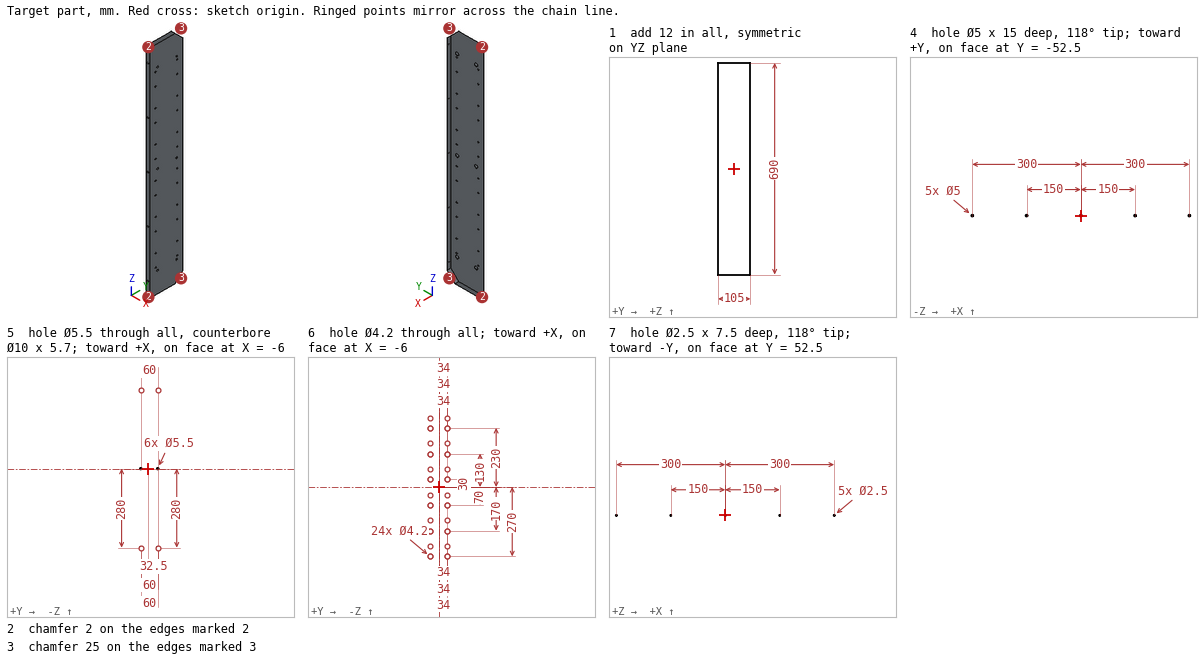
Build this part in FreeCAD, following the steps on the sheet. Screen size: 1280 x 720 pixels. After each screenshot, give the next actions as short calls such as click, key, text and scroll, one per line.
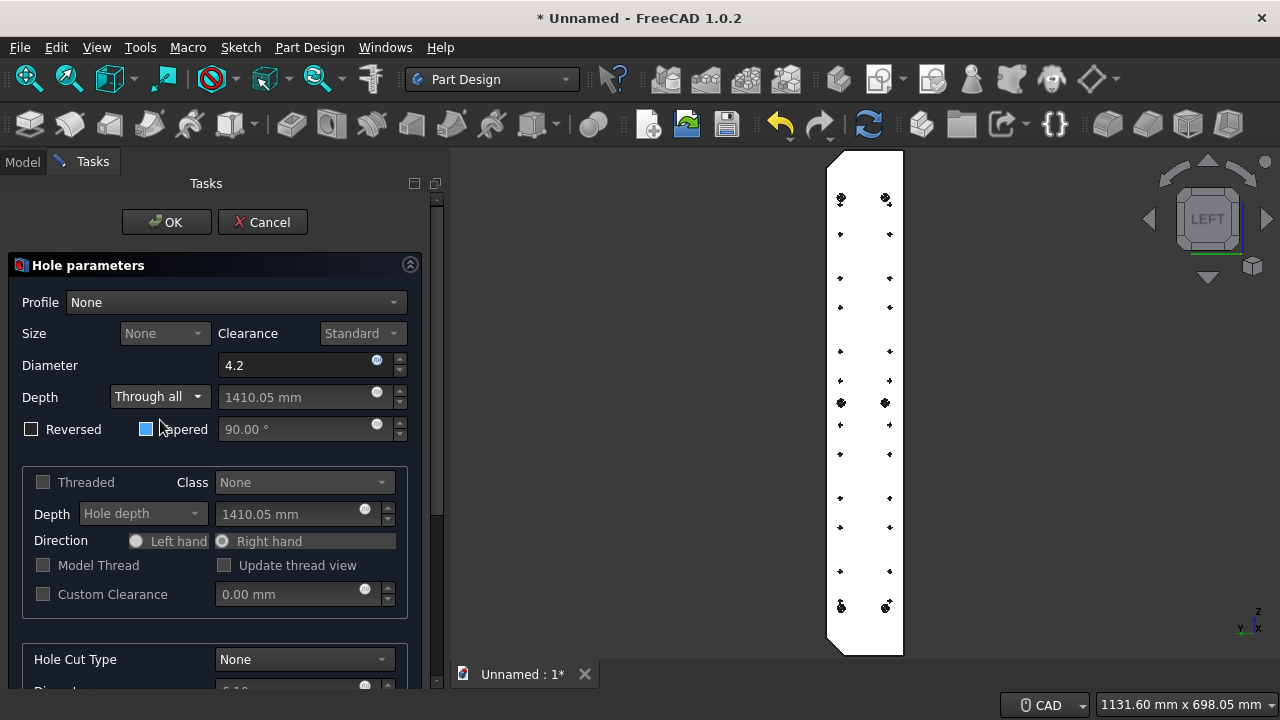
click(167, 222)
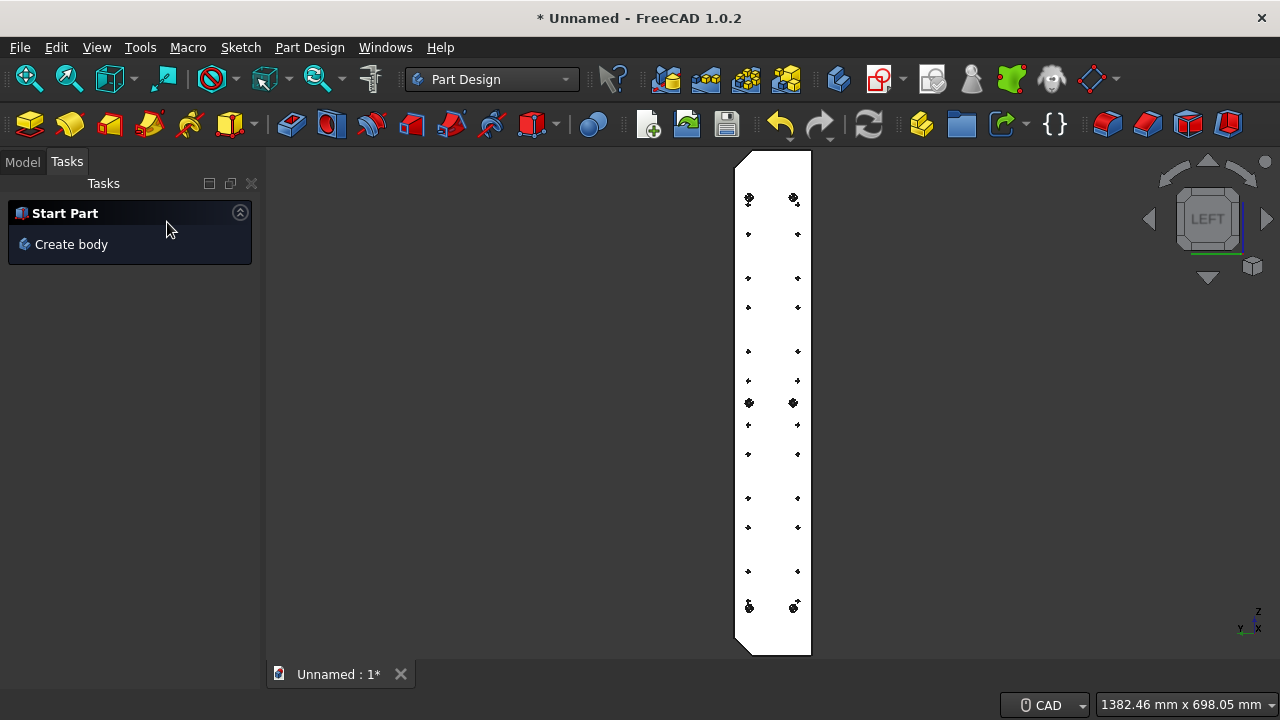
key(4)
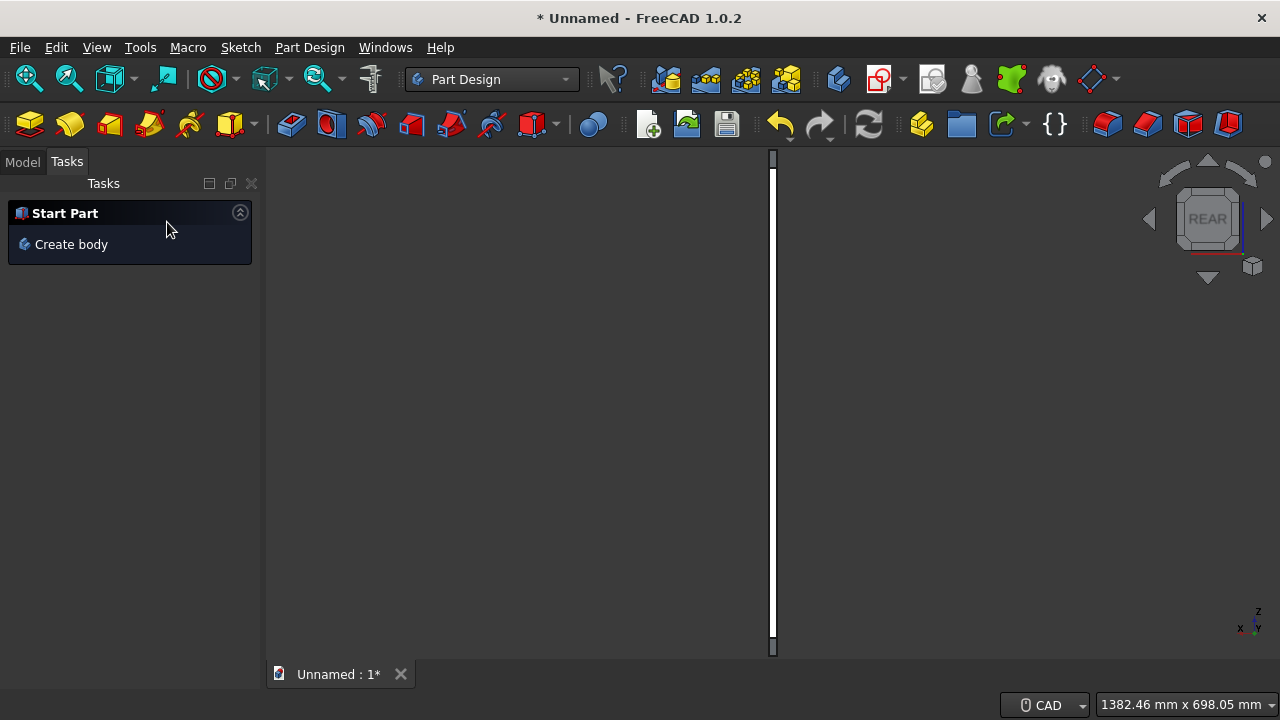
scroll(773, 402, up, 6)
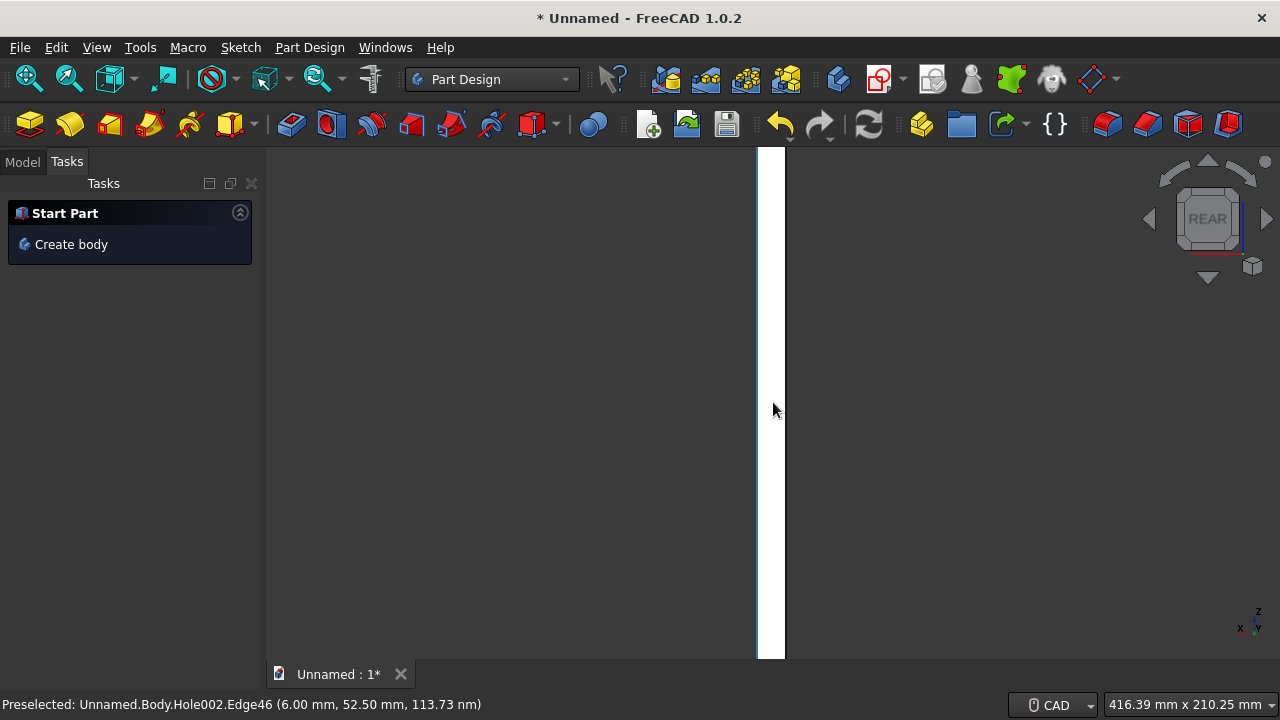
click(772, 403)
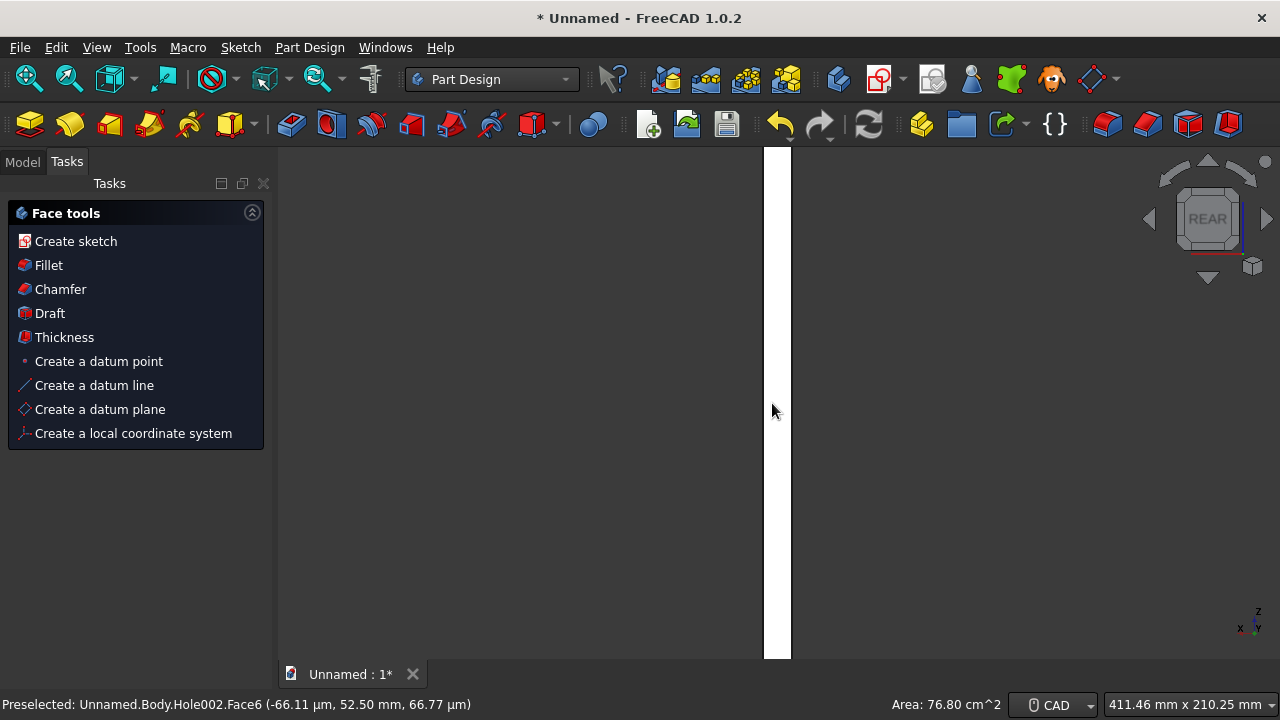
click(880, 80)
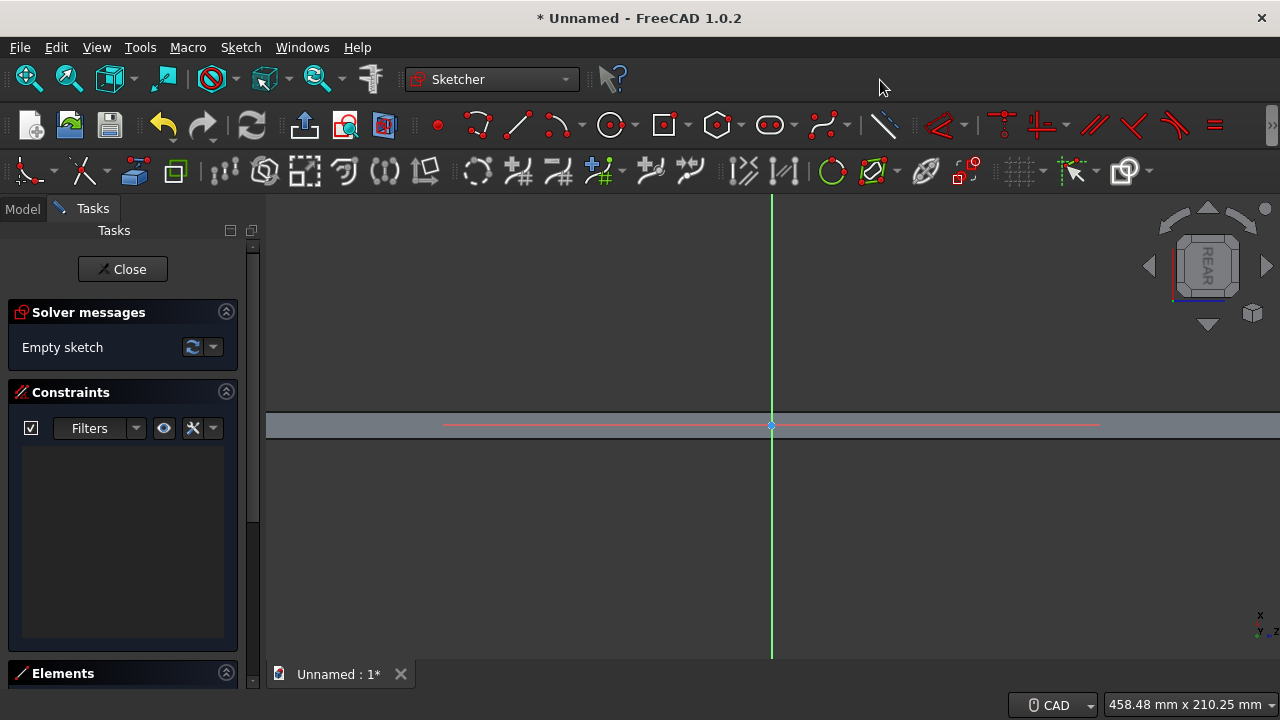
scroll(649, 427, down, 4)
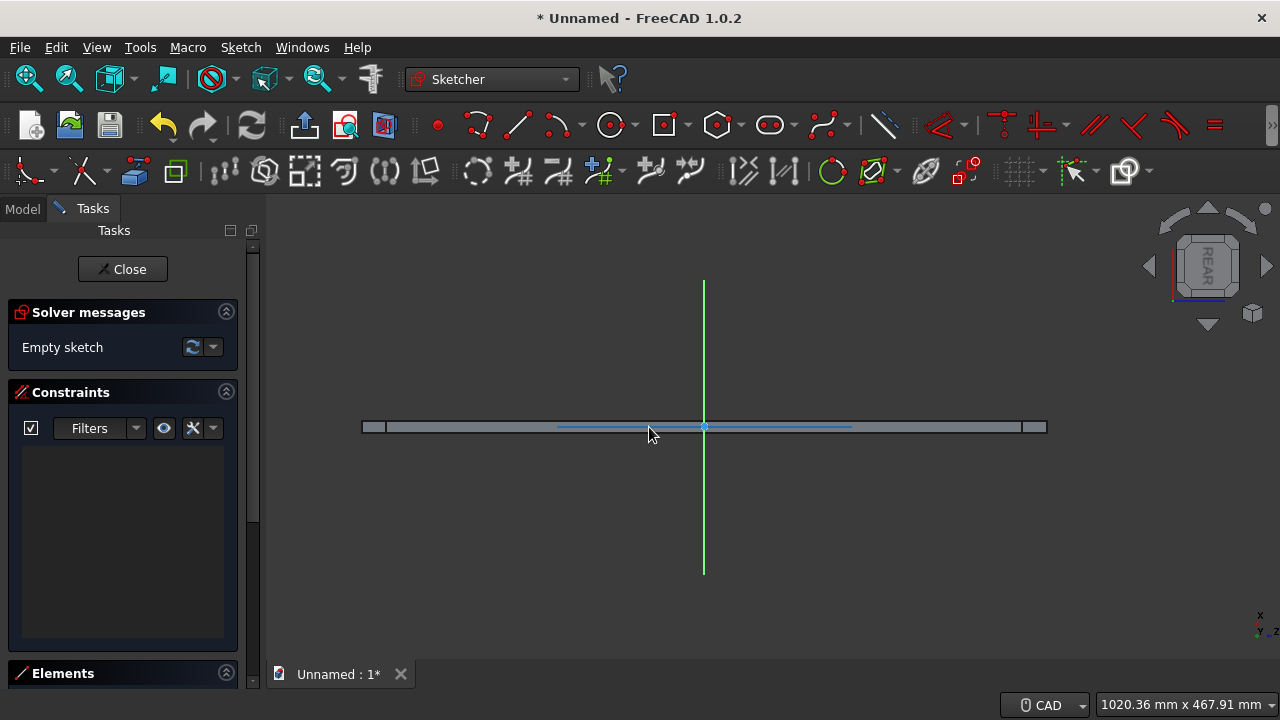
click(612, 126)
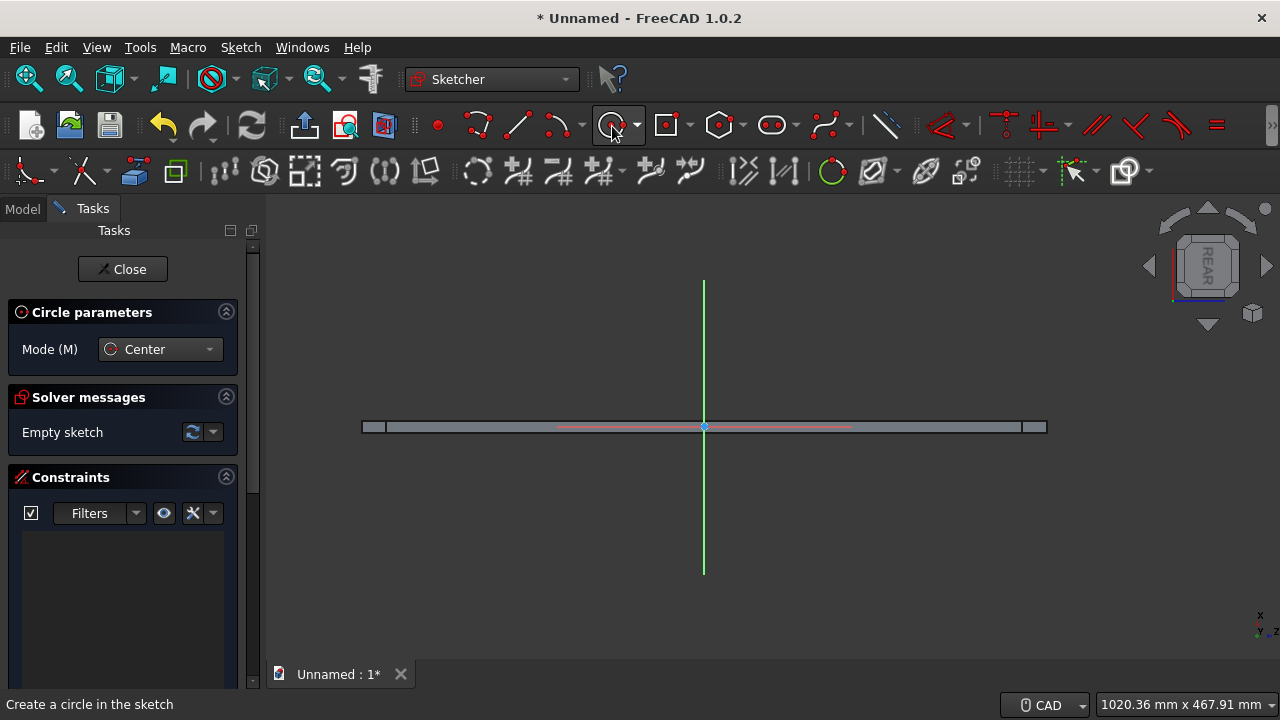
scroll(1003, 427, up, 15)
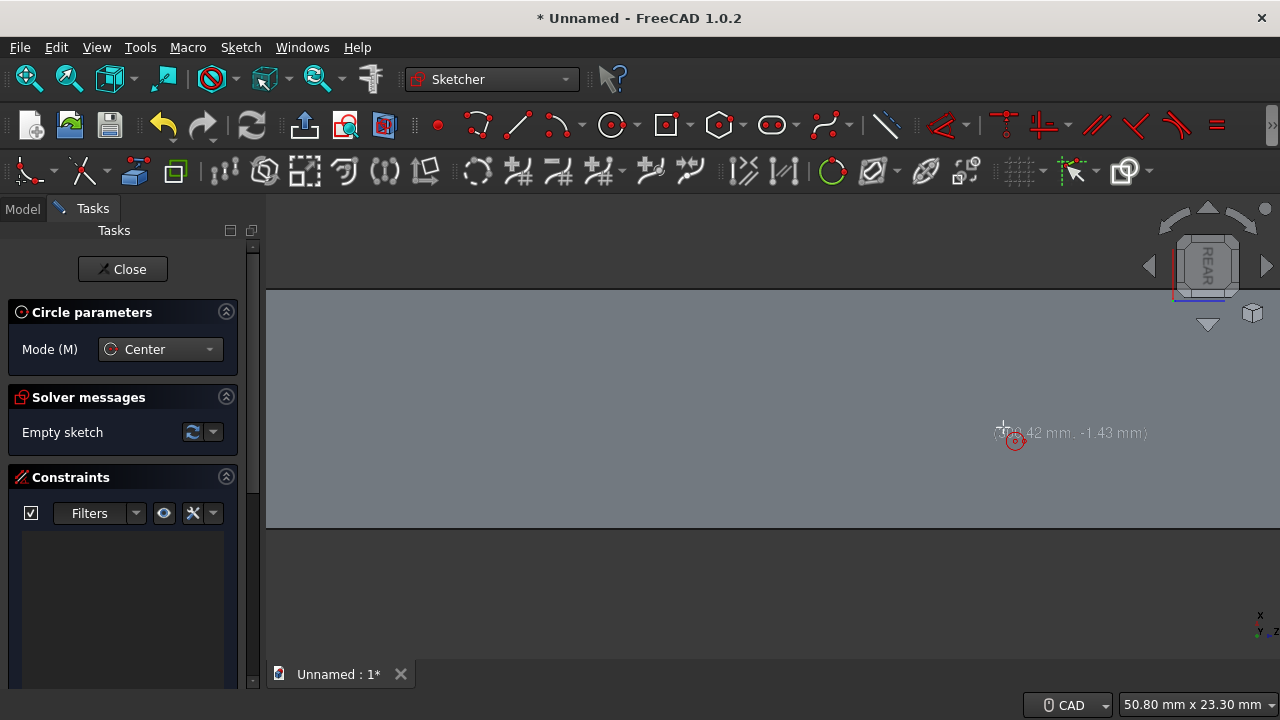
scroll(1004, 427, down, 15)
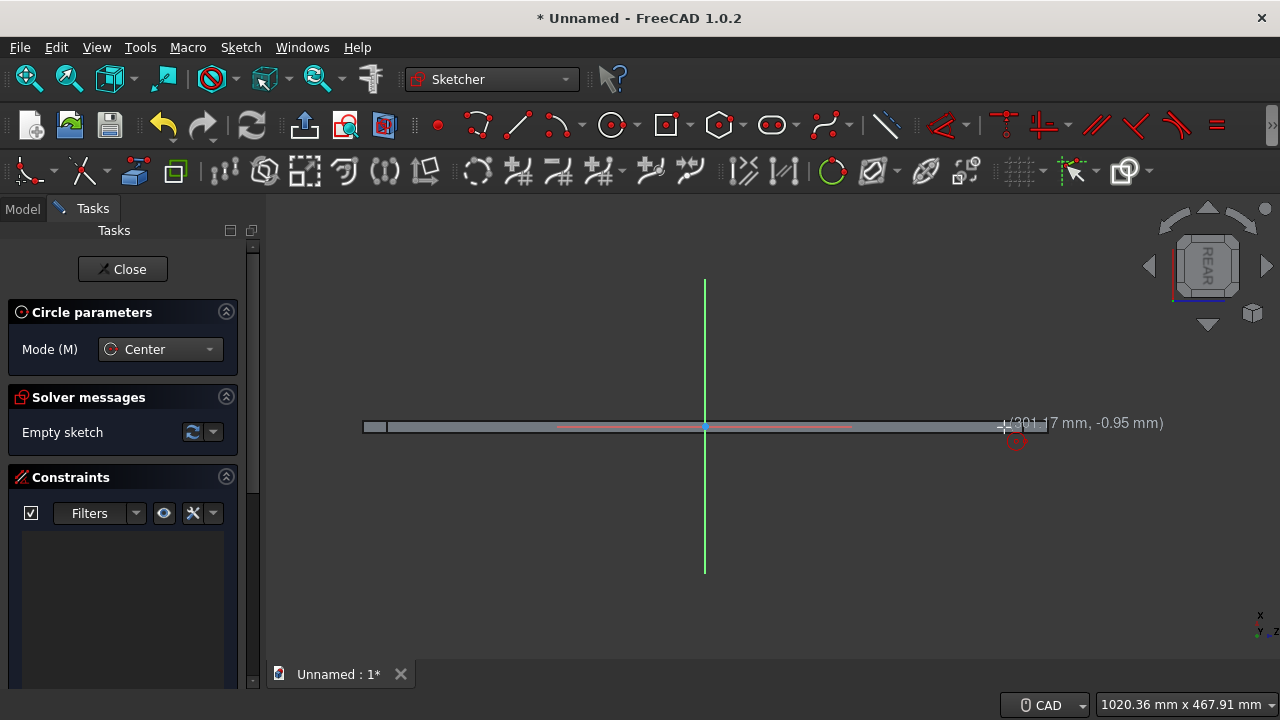
click(1004, 427)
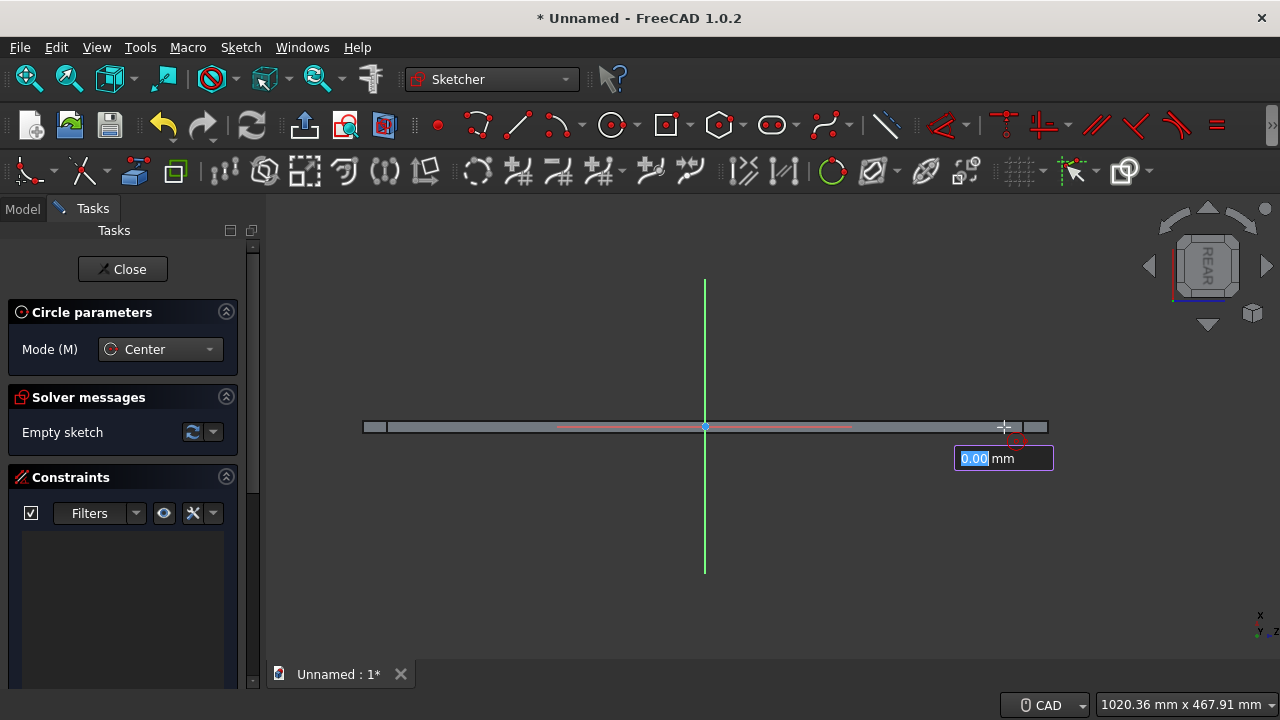
scroll(1003, 428, up, 14)
move(994, 416)